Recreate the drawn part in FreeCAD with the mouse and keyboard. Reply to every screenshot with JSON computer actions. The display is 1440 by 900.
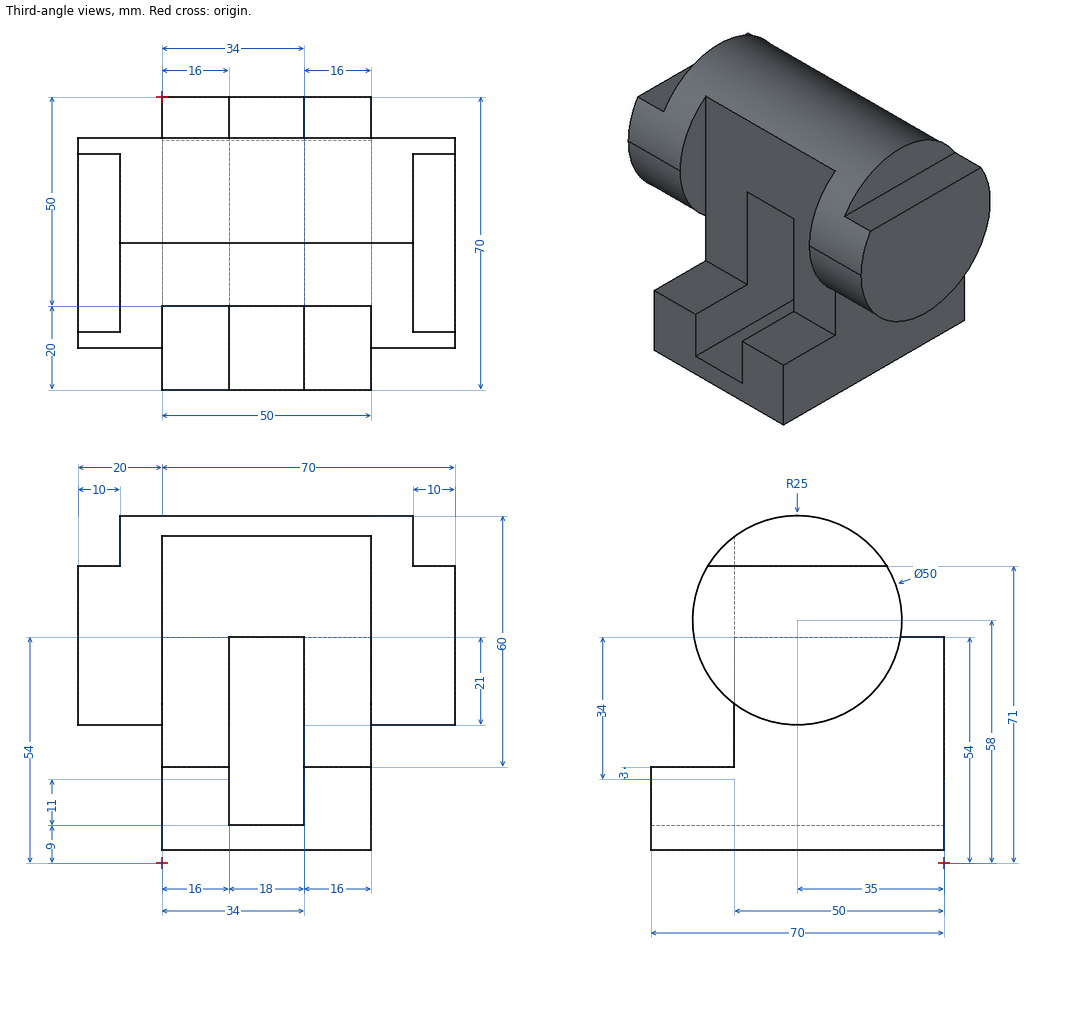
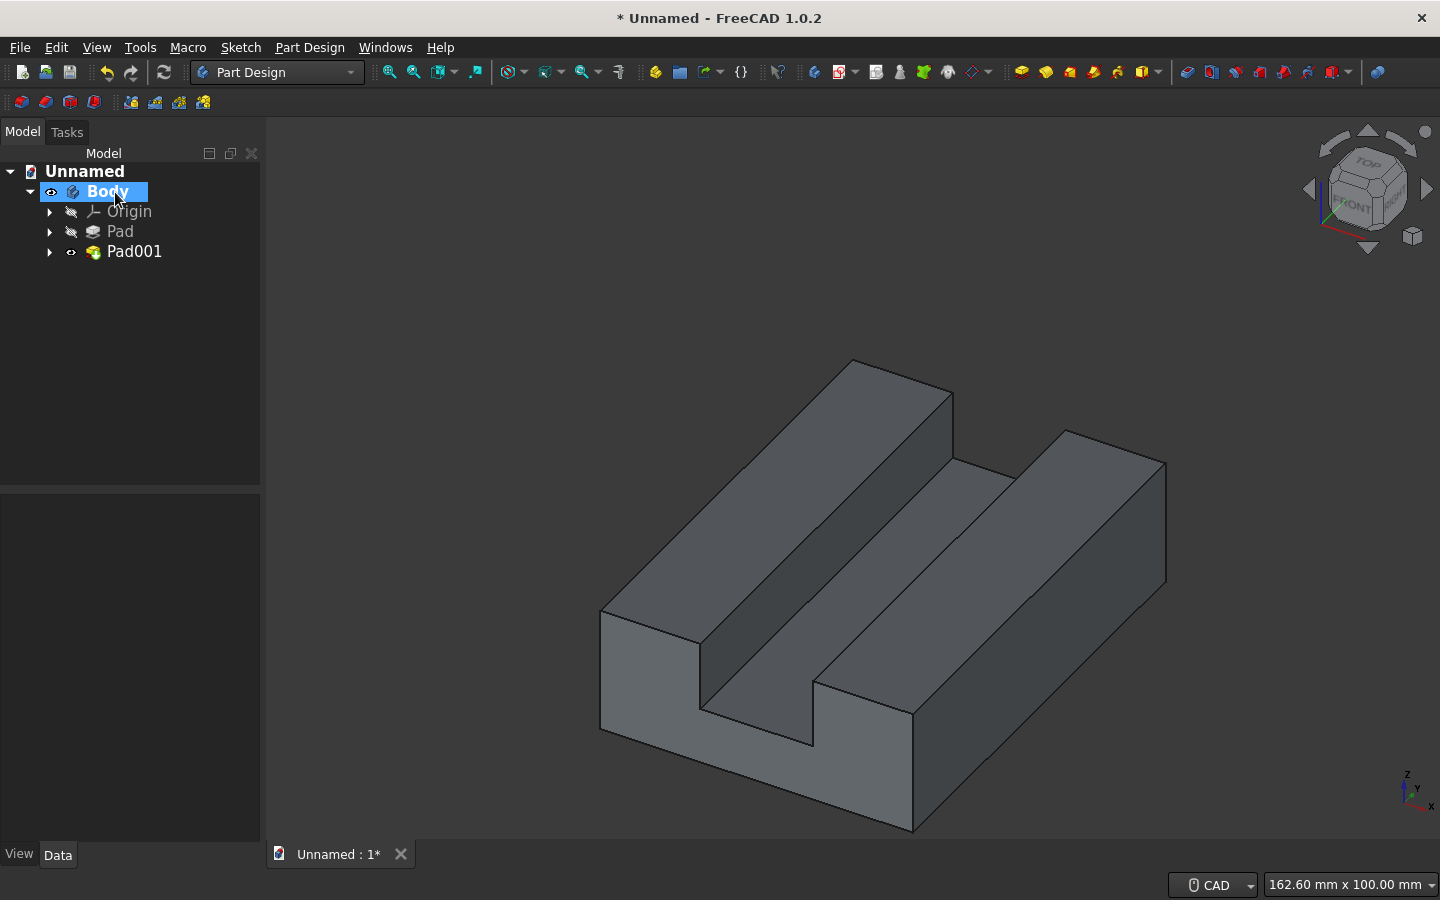
{"action": "left_click", "coordinate": [840, 72]}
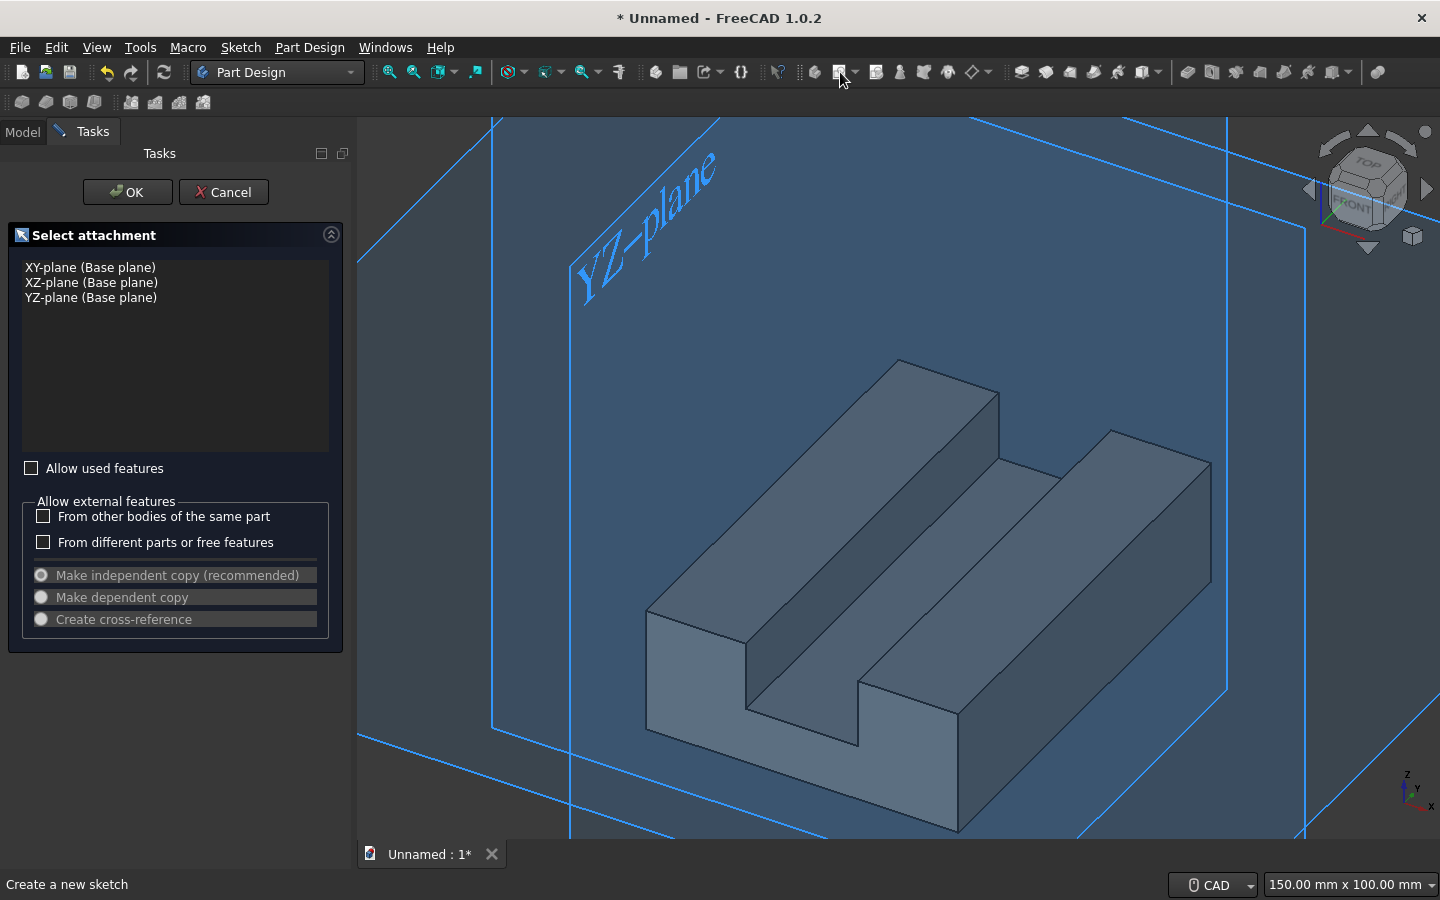
{"action": "left_click", "coordinate": [82, 298]}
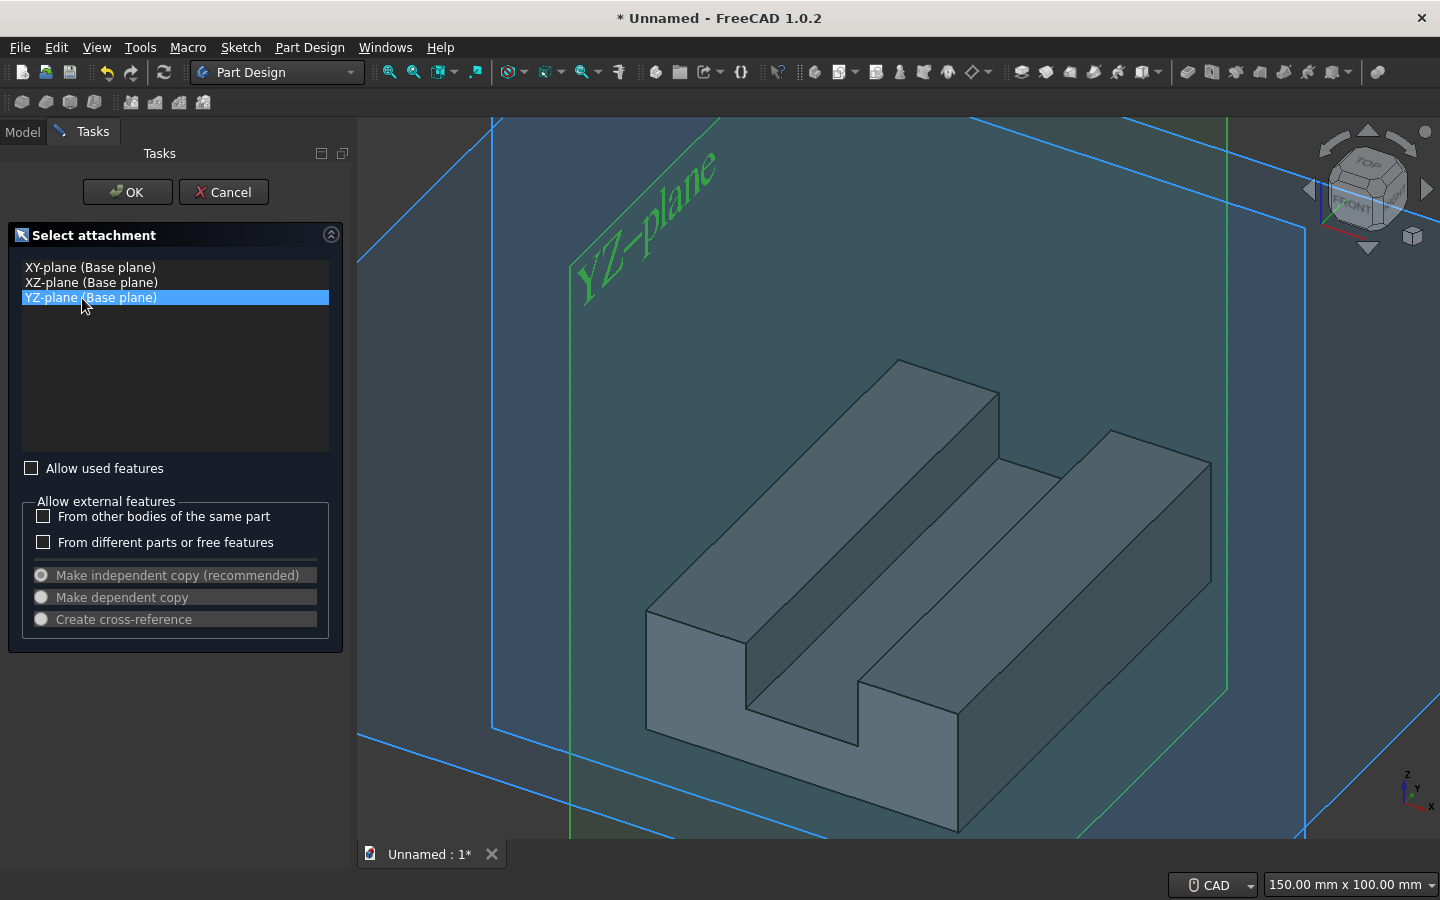
{"action": "left_click", "coordinate": [128, 192]}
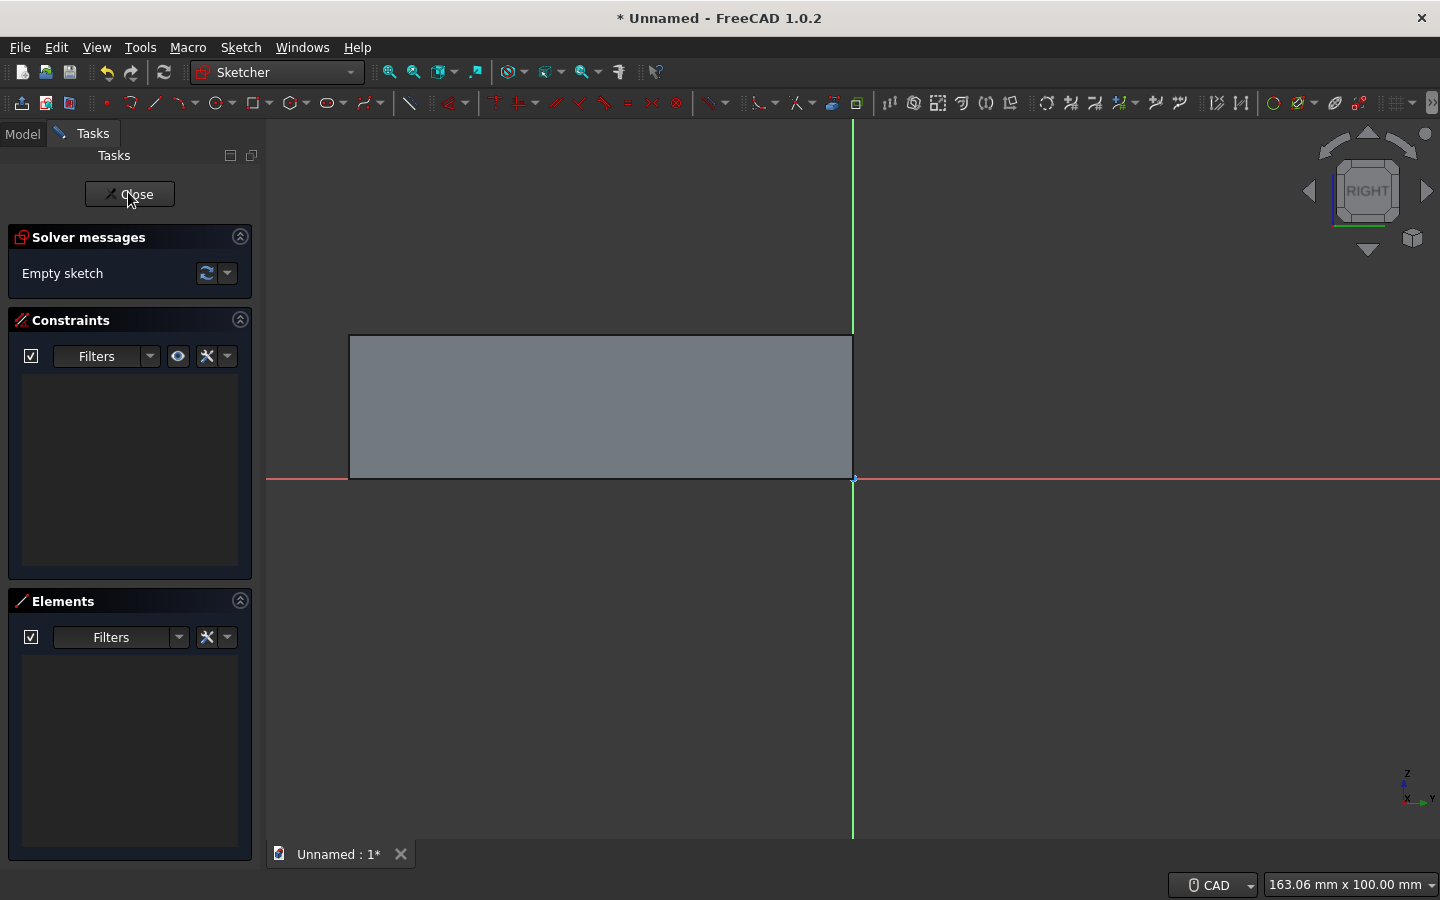
{"action": "left_click", "coordinate": [70, 104]}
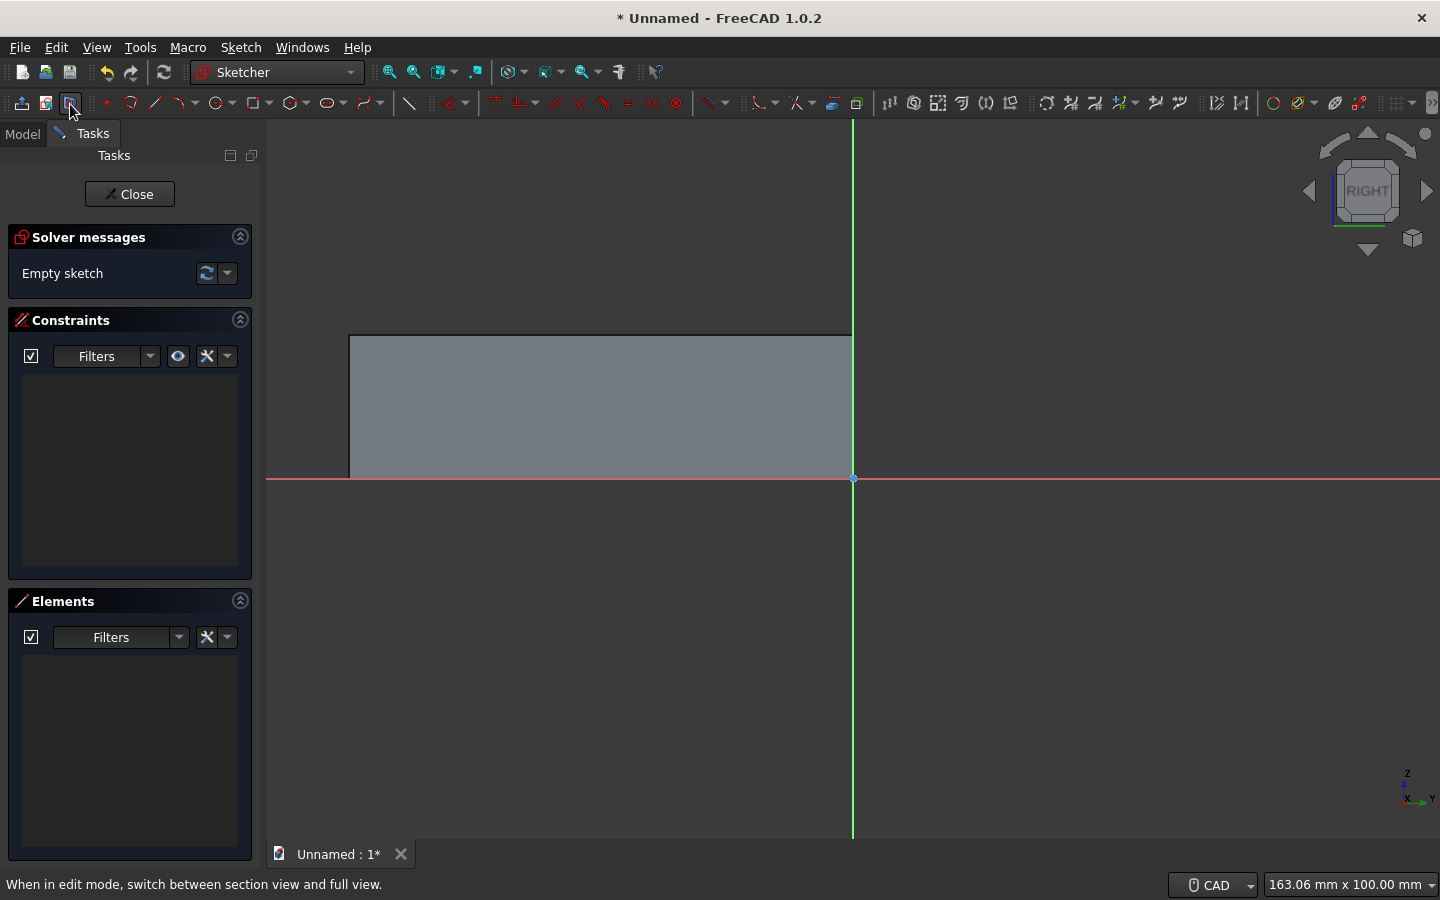
{"action": "scroll", "coordinate": [1275, 811], "scroll_direction": "down", "scroll_amount": 1}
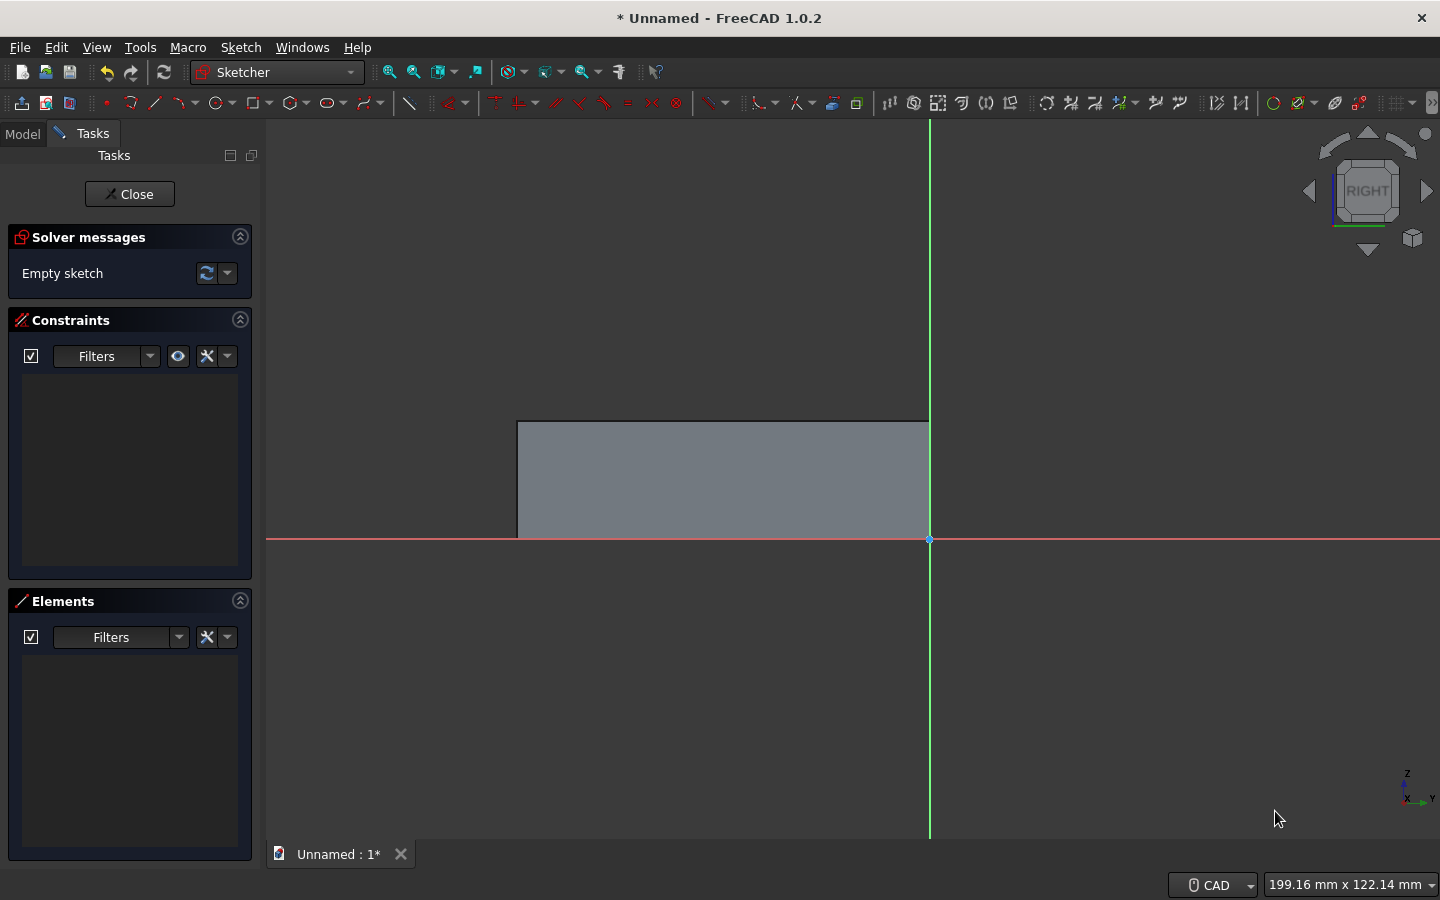
{"action": "scroll", "coordinate": [778, 179], "scroll_direction": "up", "scroll_amount": 2}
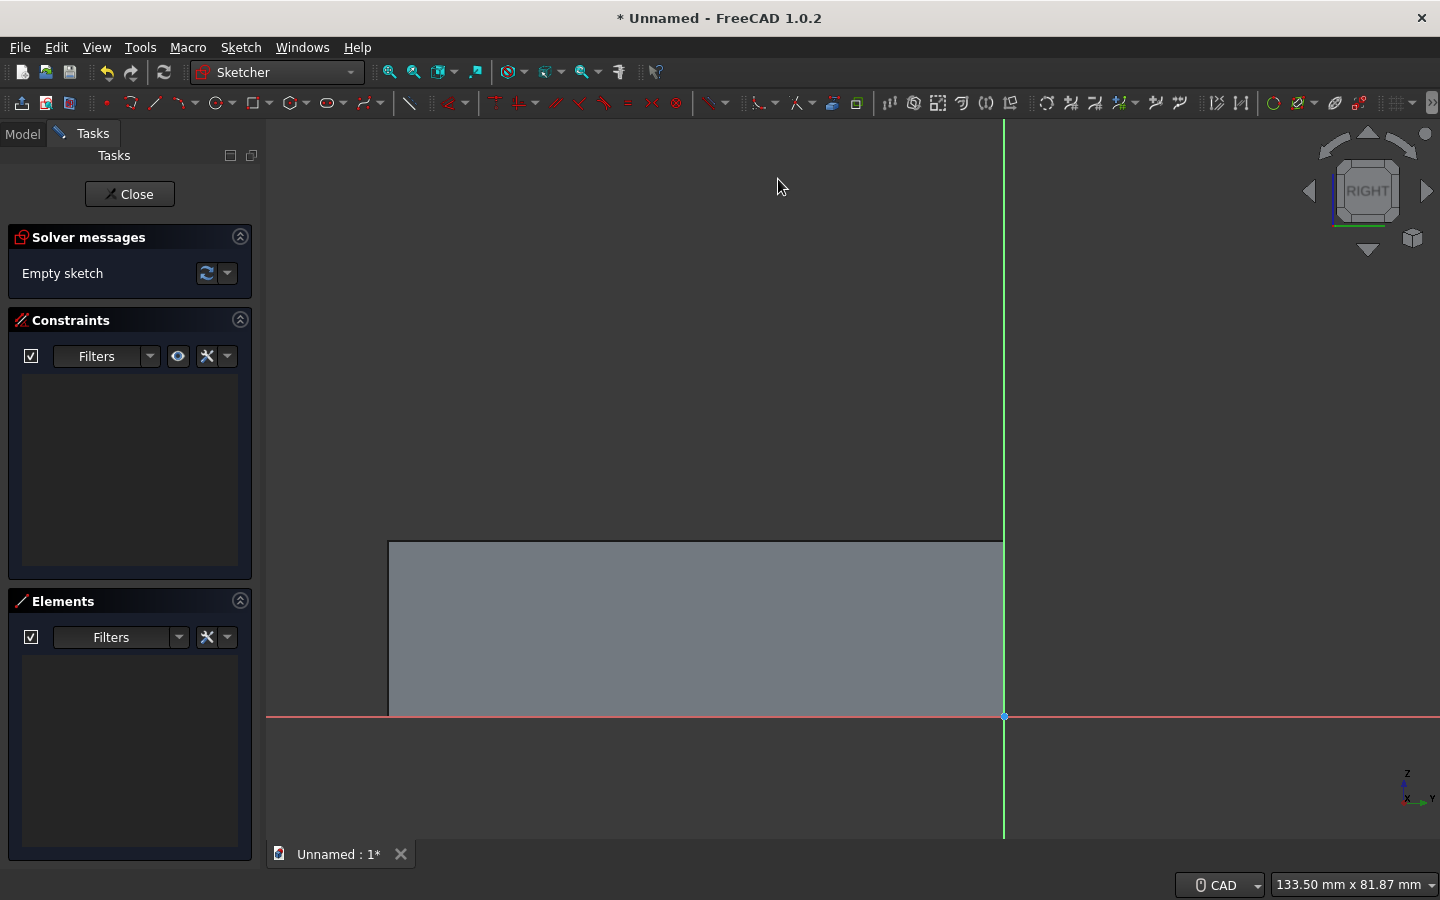
{"action": "left_click", "coordinate": [254, 104]}